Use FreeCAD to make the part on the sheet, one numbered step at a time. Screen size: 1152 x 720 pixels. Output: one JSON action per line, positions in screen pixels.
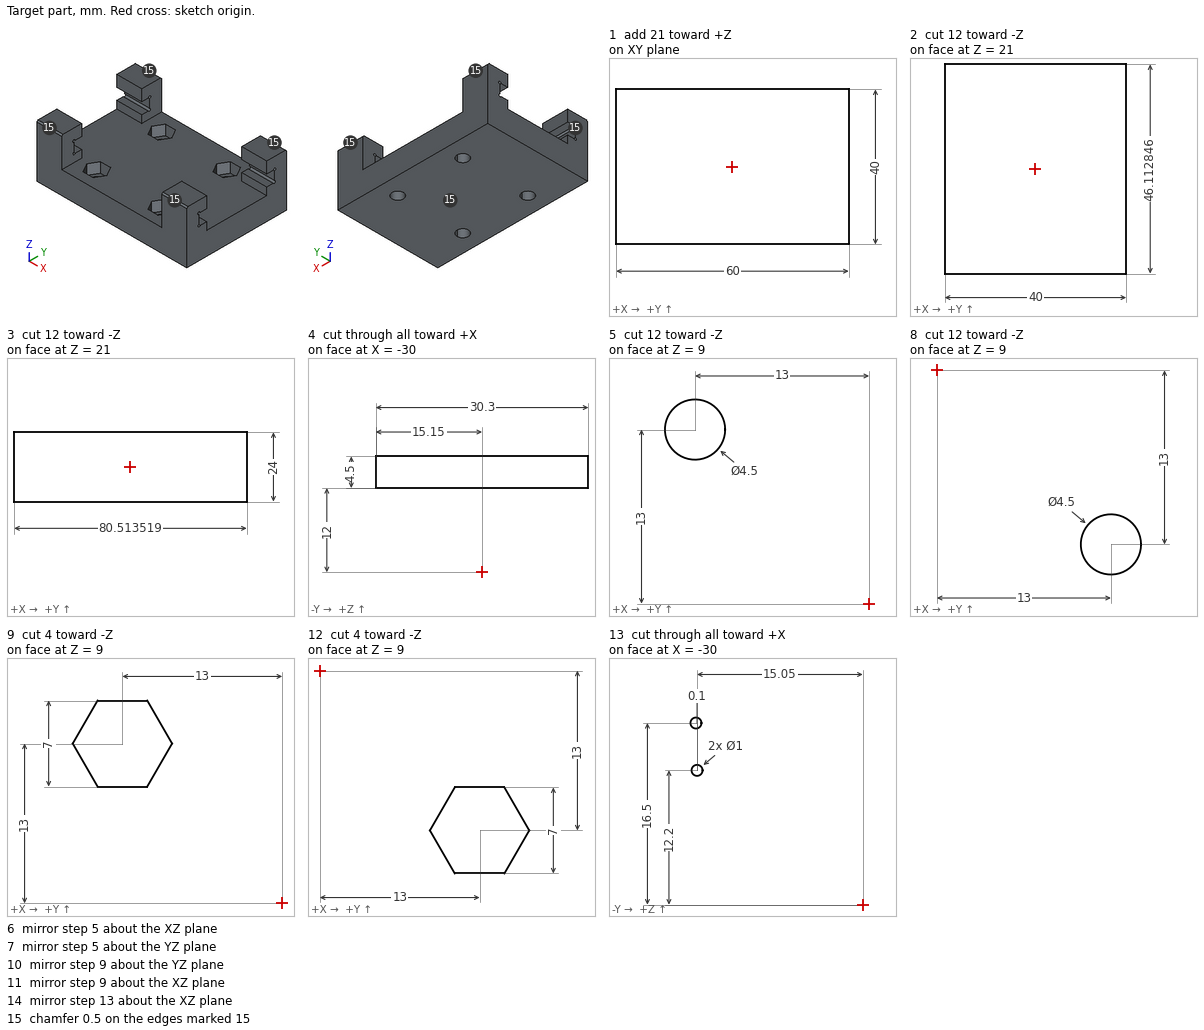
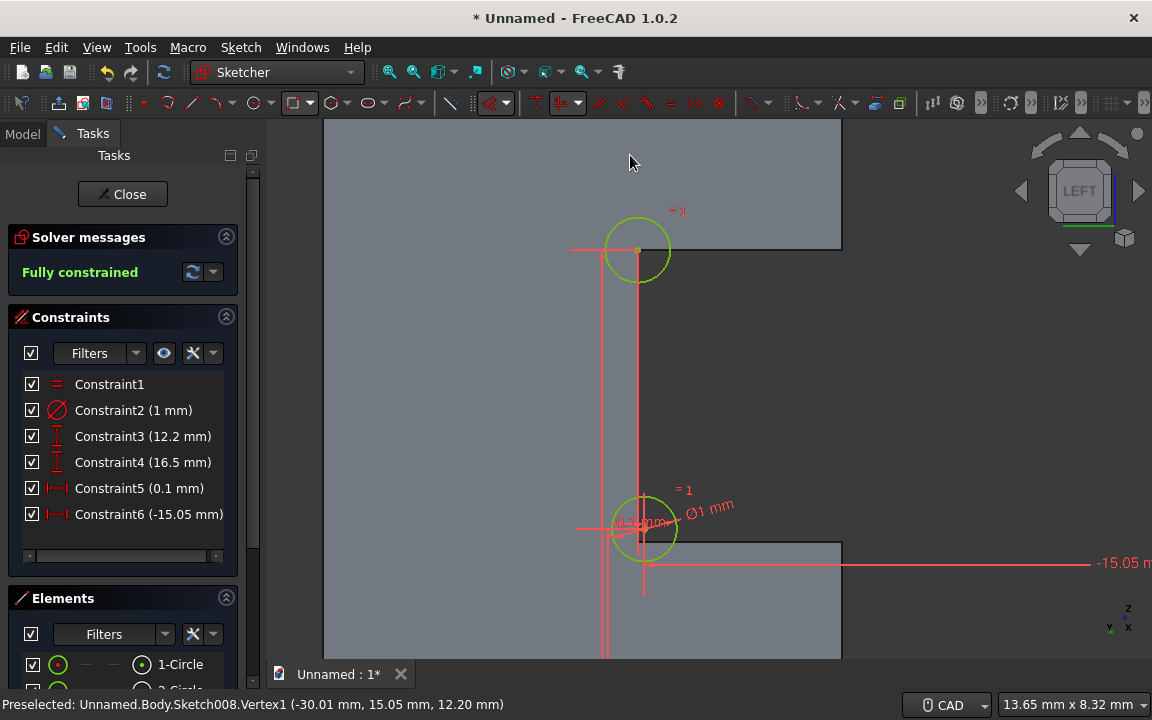
{"action": "left_click", "coordinate": [123, 194]}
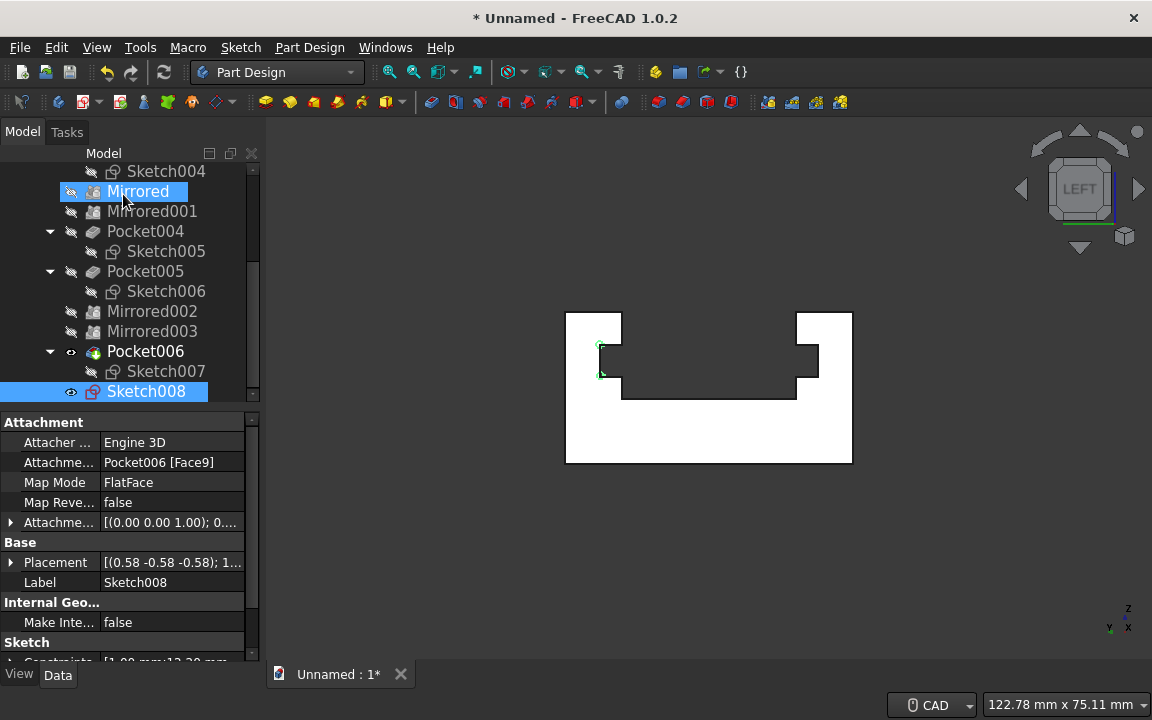
{"action": "left_click", "coordinate": [432, 102]}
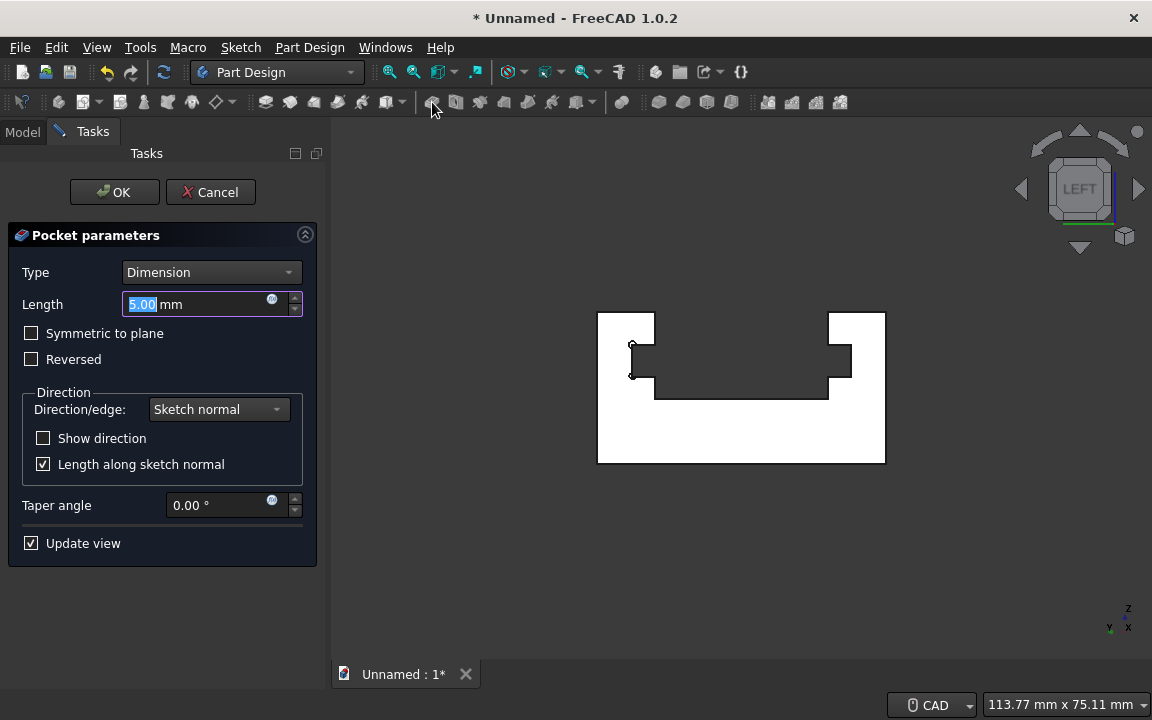
{"action": "left_click", "coordinate": [212, 272]}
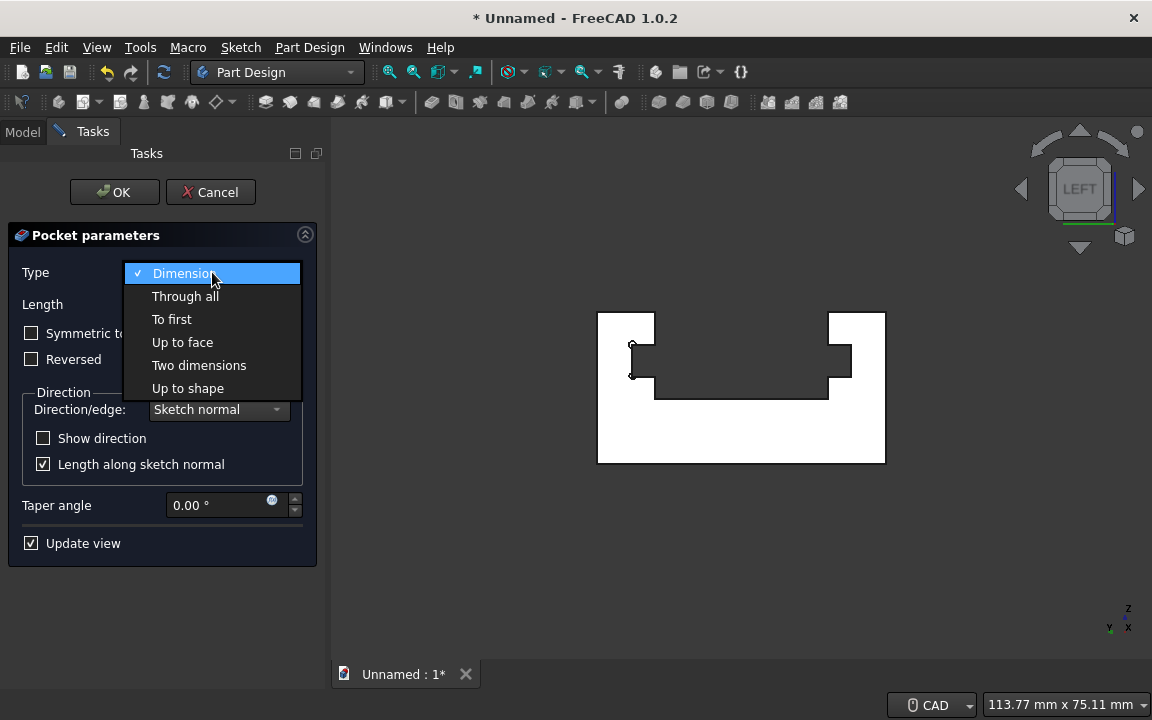
{"action": "left_click", "coordinate": [212, 296]}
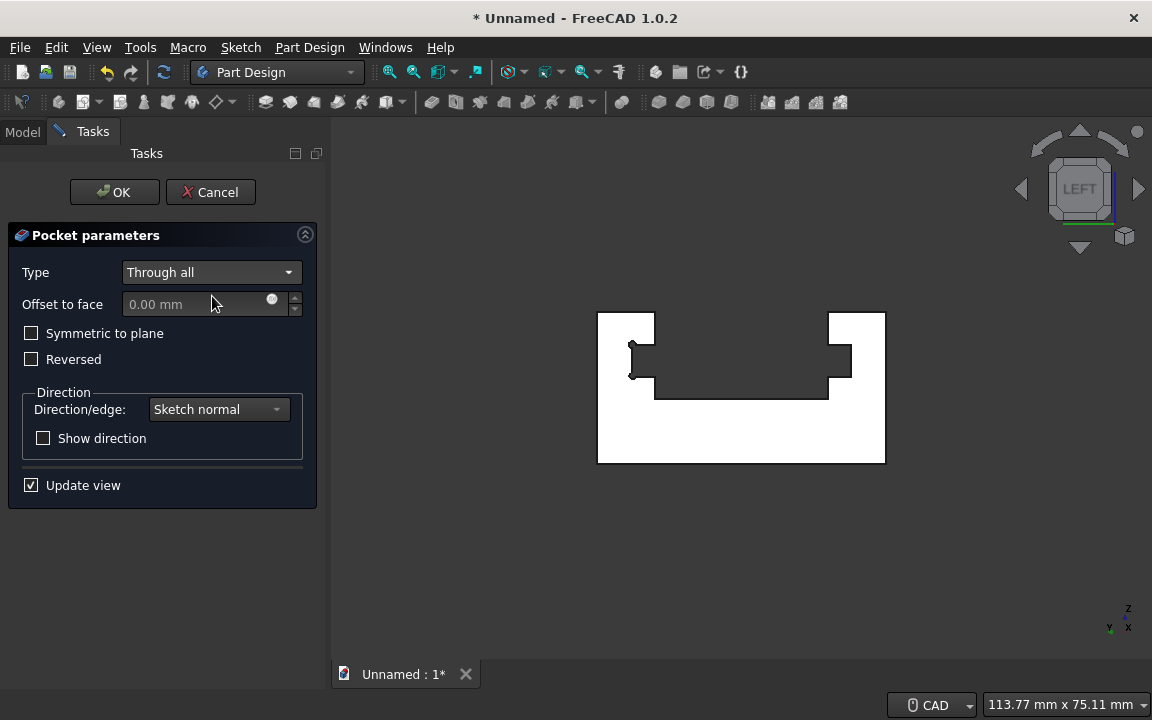
{"action": "left_click", "coordinate": [115, 192]}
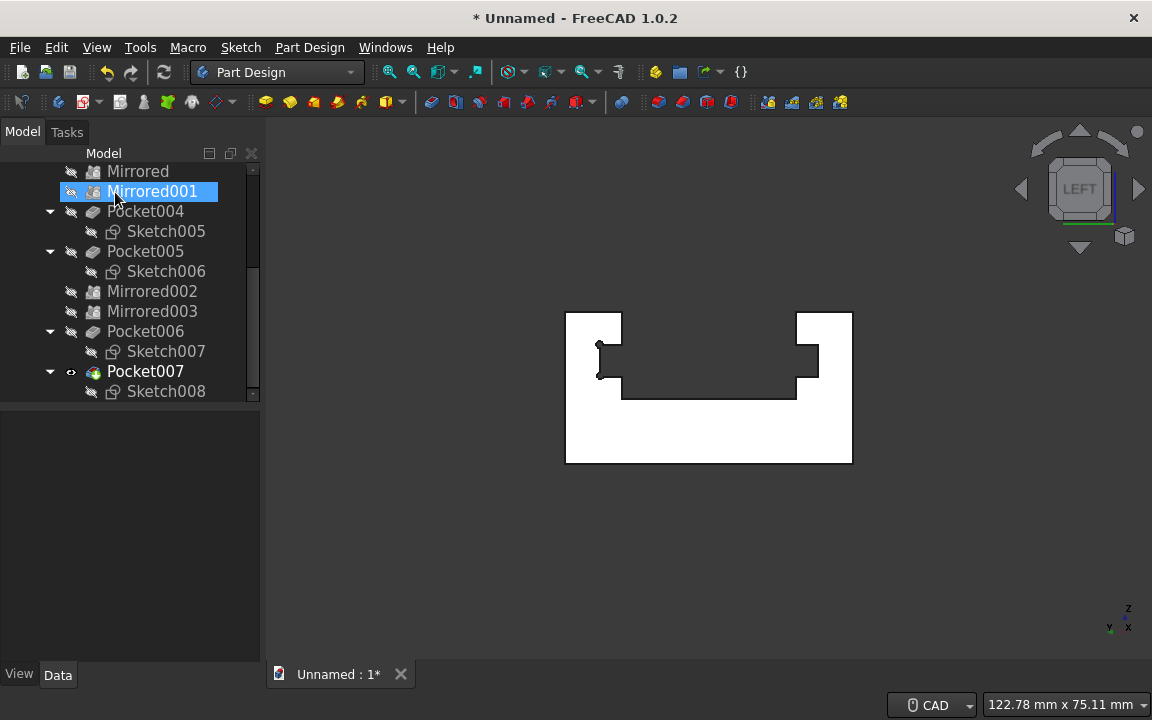
{"action": "left_click", "coordinate": [390, 72]}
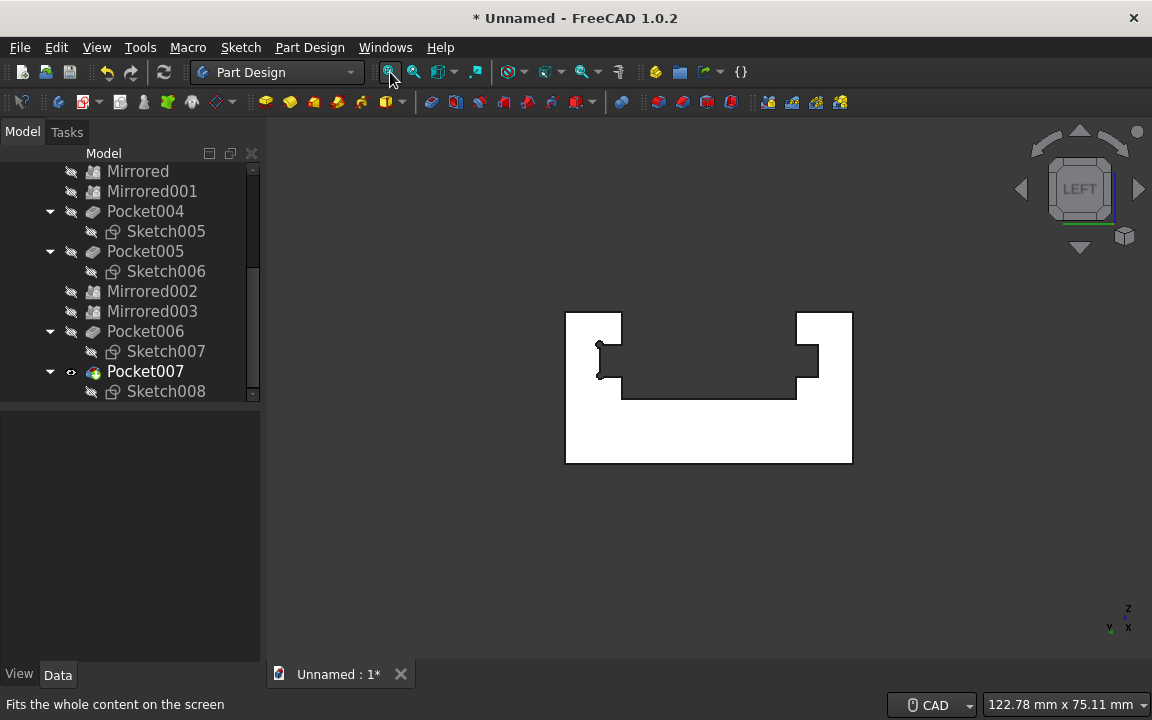
{"action": "left_click", "coordinate": [116, 372]}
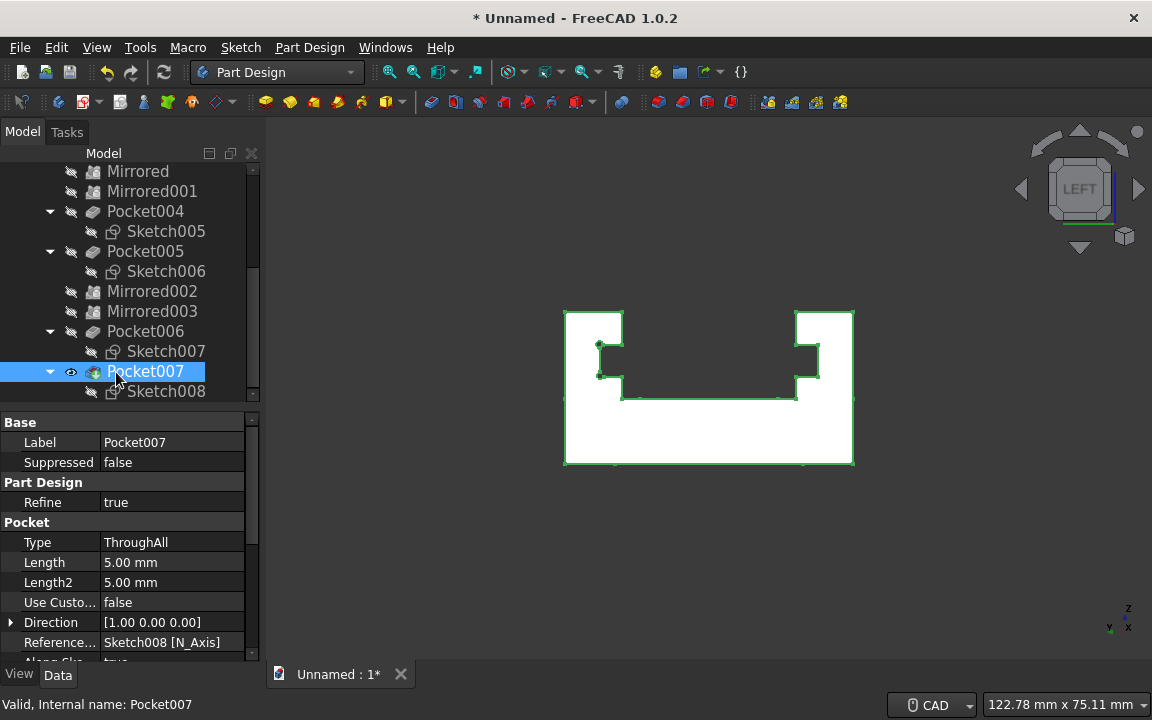
{"action": "left_click", "coordinate": [768, 102]}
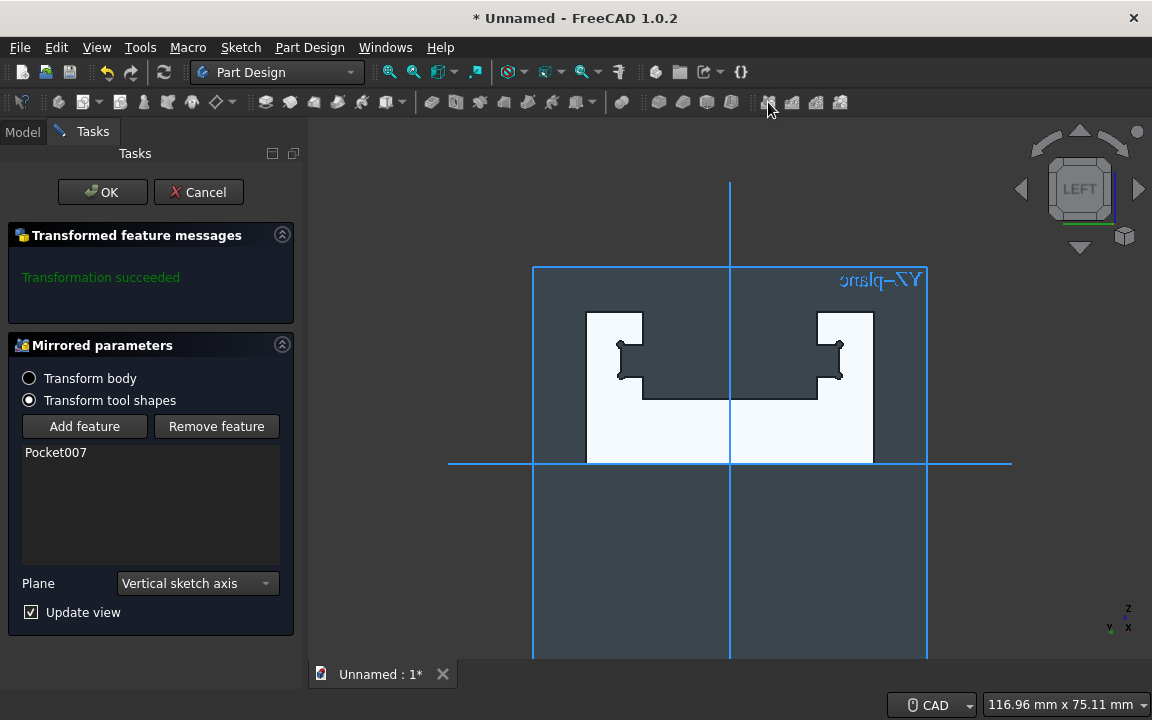
{"action": "left_click", "coordinate": [198, 584]}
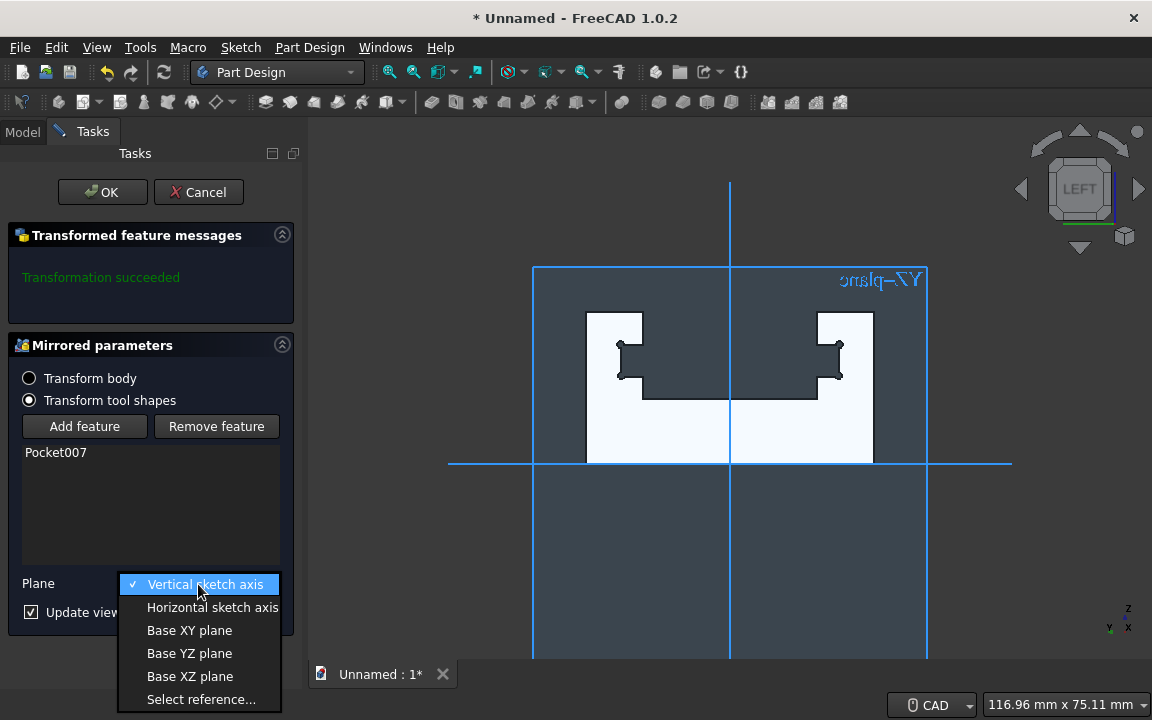
{"action": "left_click", "coordinate": [198, 676]}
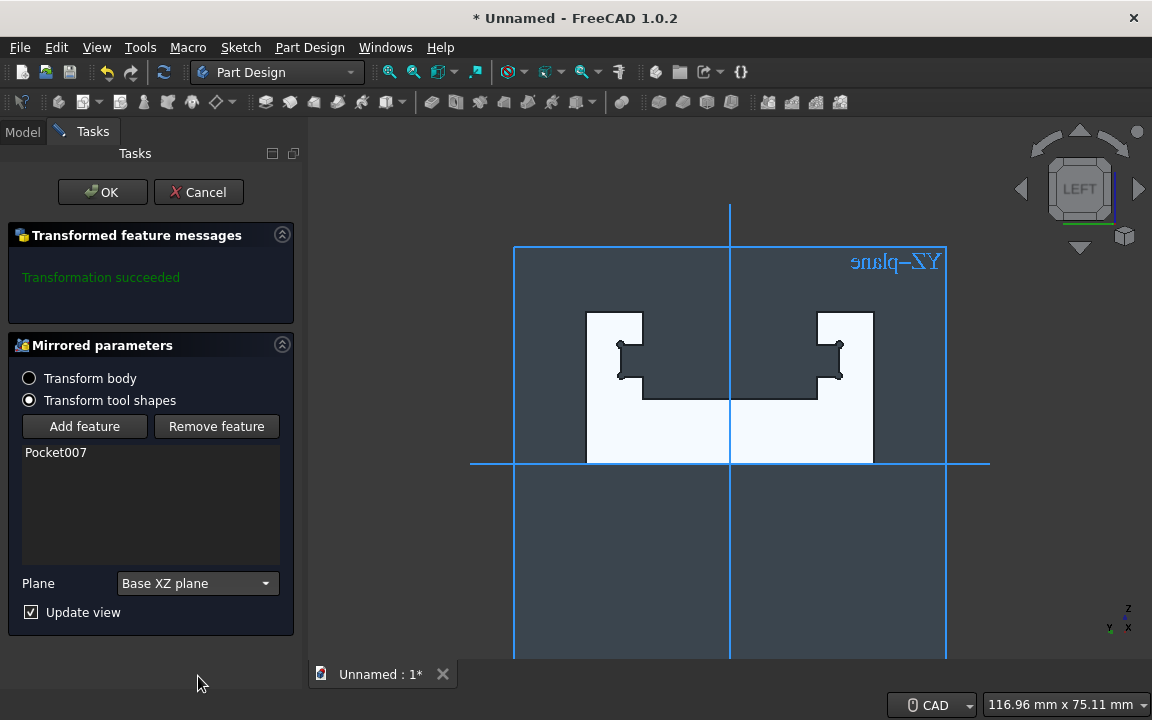
{"action": "left_click", "coordinate": [103, 192]}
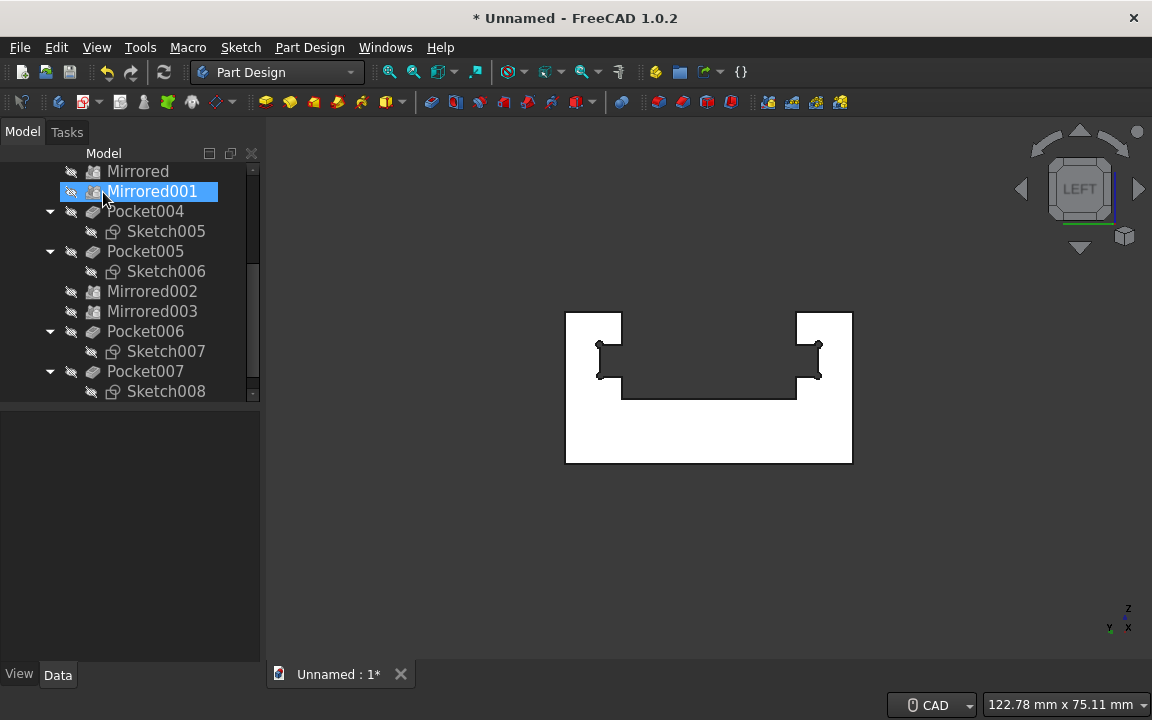
{"action": "left_click", "coordinate": [390, 72]}